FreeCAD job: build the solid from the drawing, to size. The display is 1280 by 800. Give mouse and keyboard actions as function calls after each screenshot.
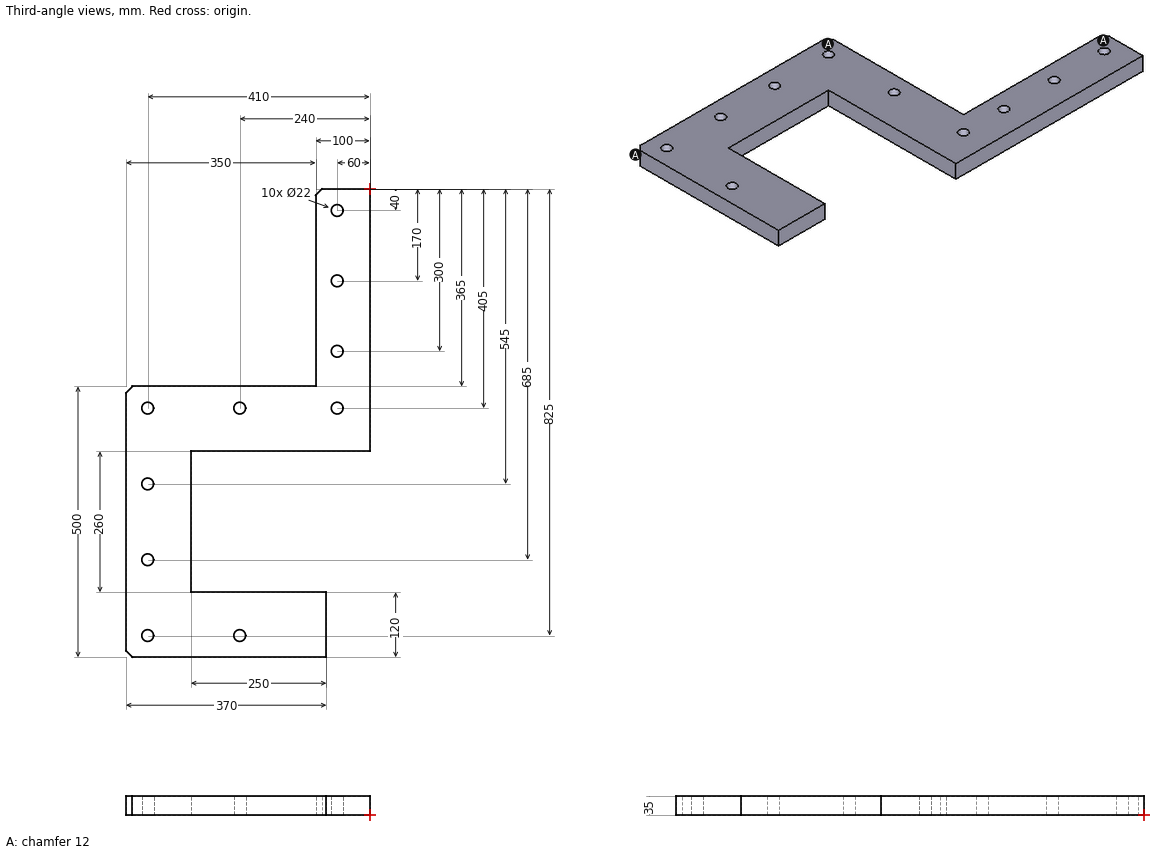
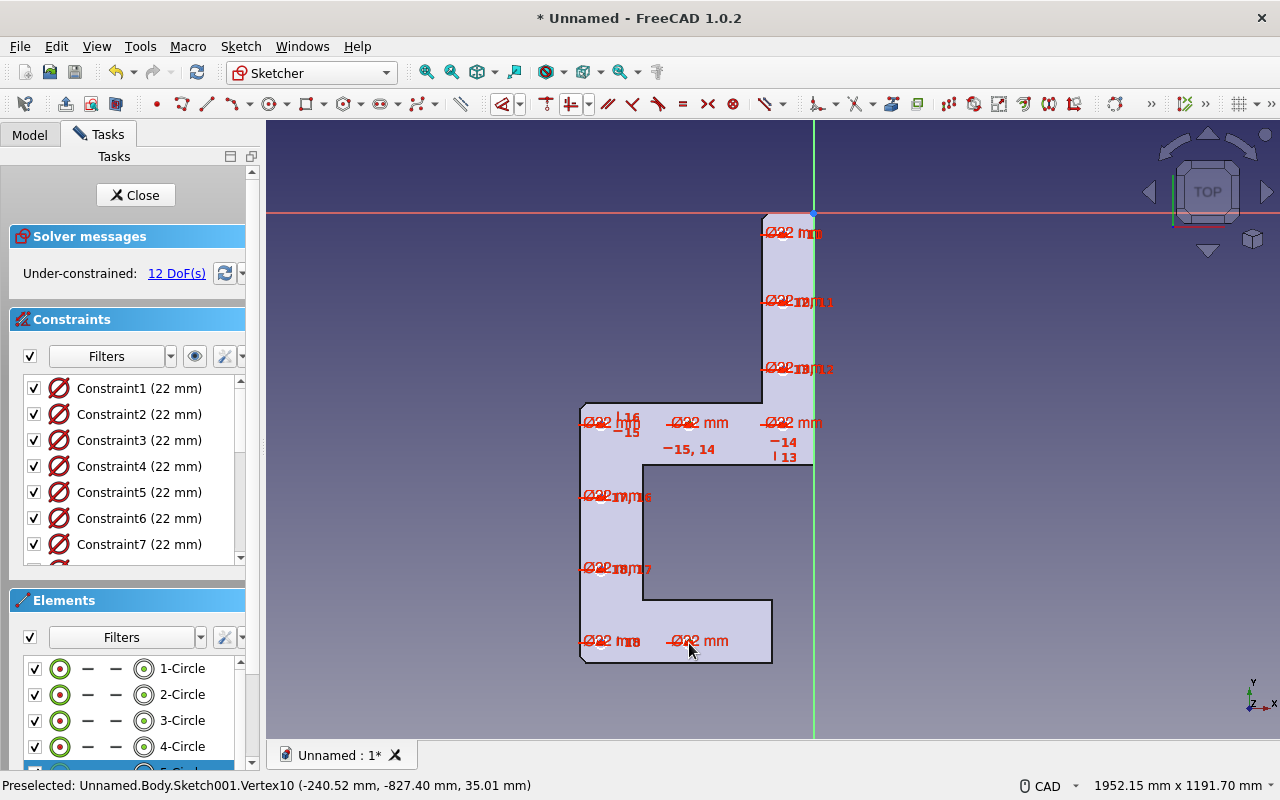
click(588, 104)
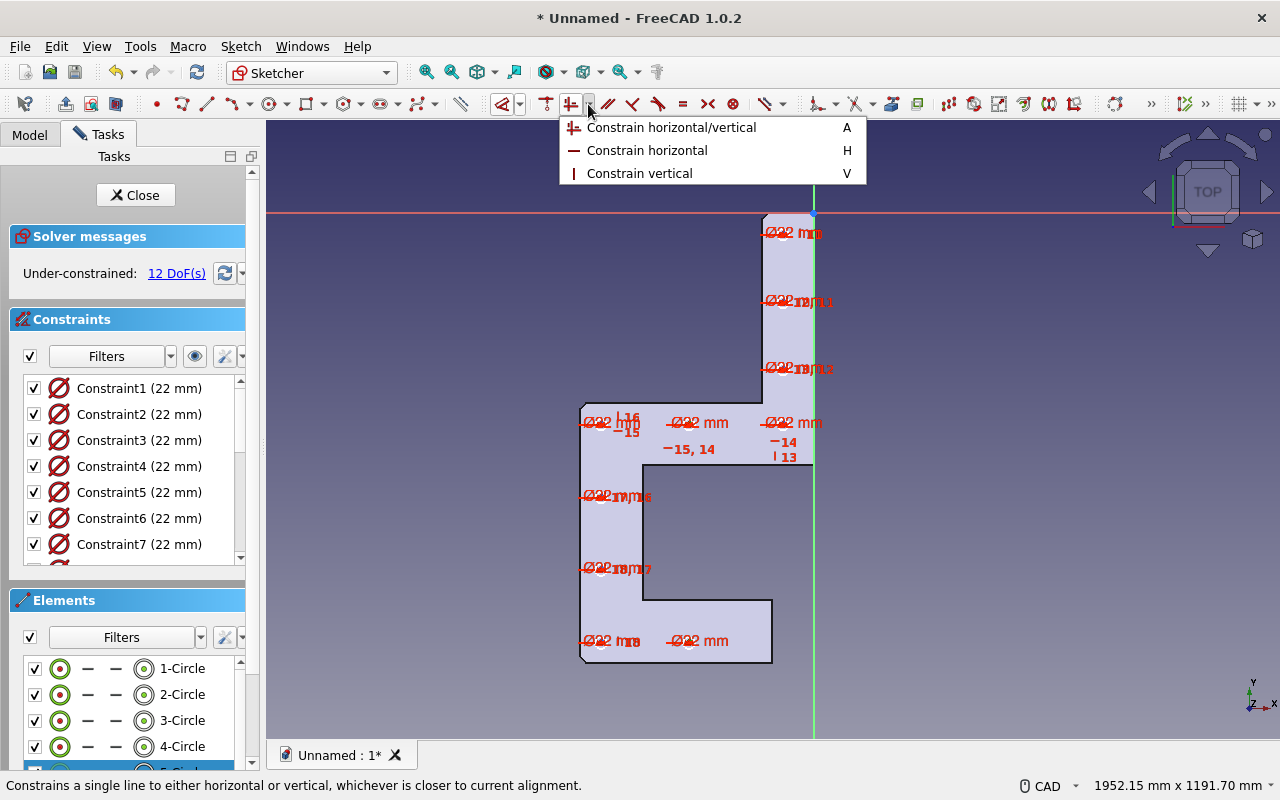
click(713, 174)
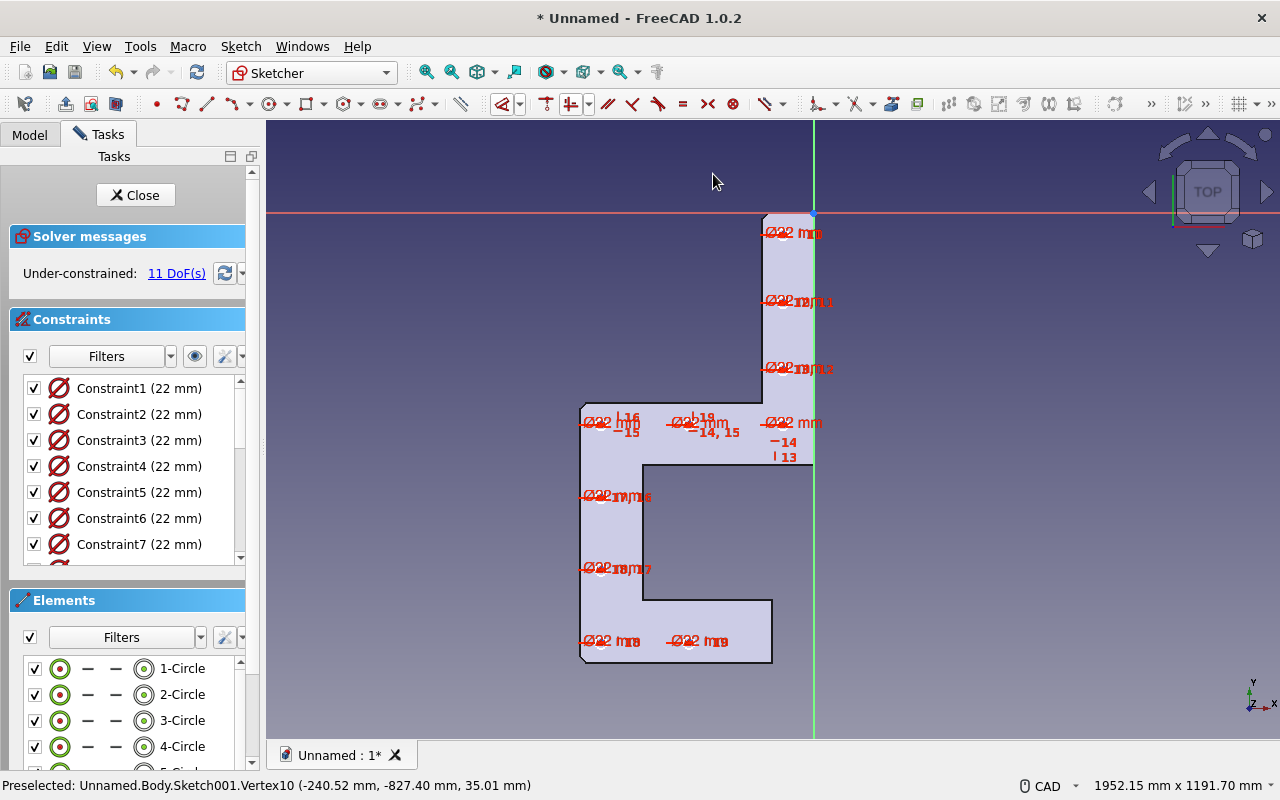
click(601, 643)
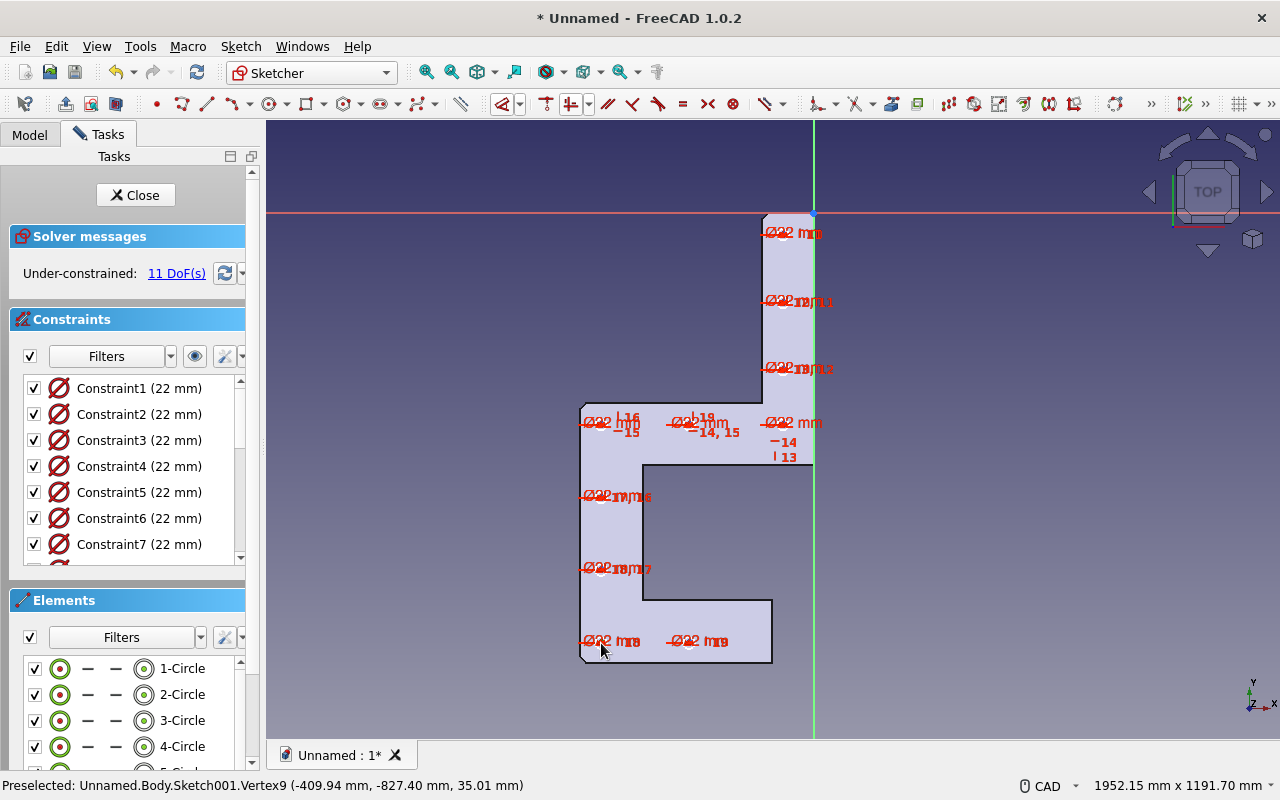
click(689, 643)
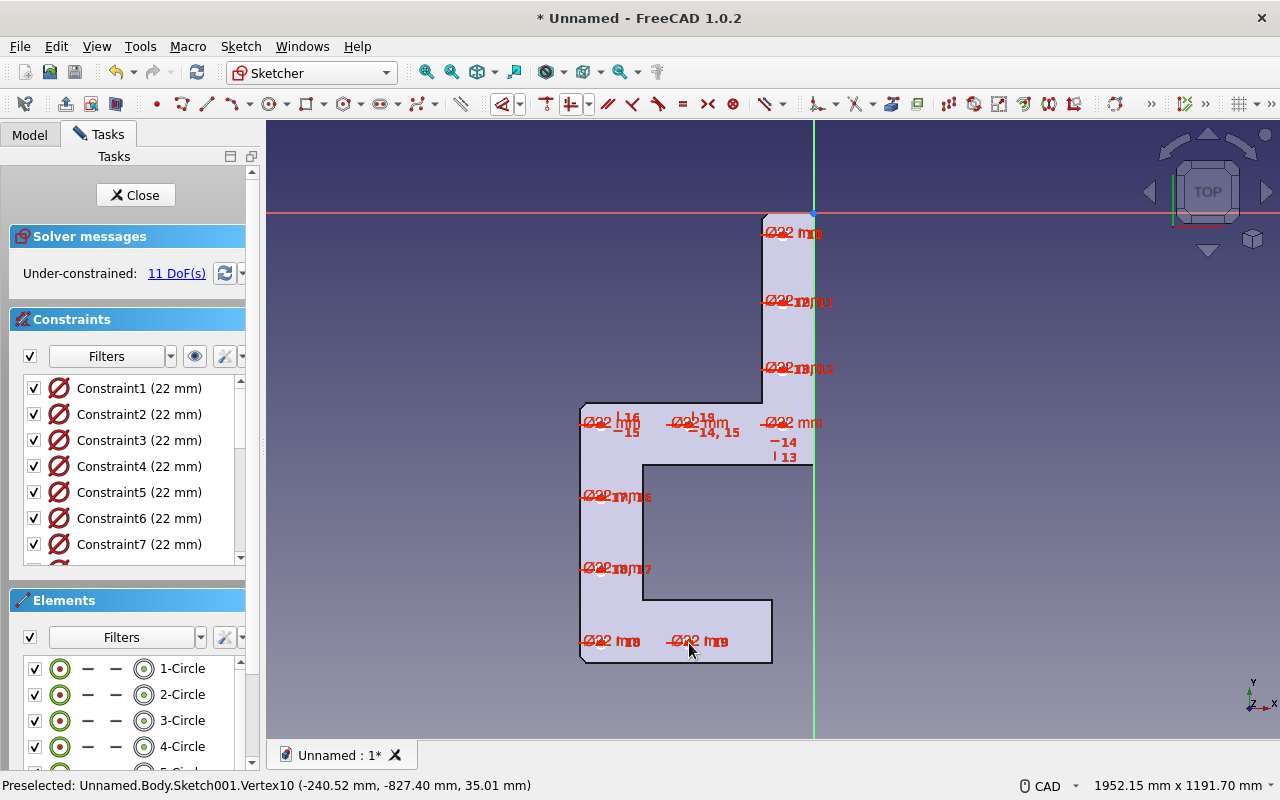
click(588, 104)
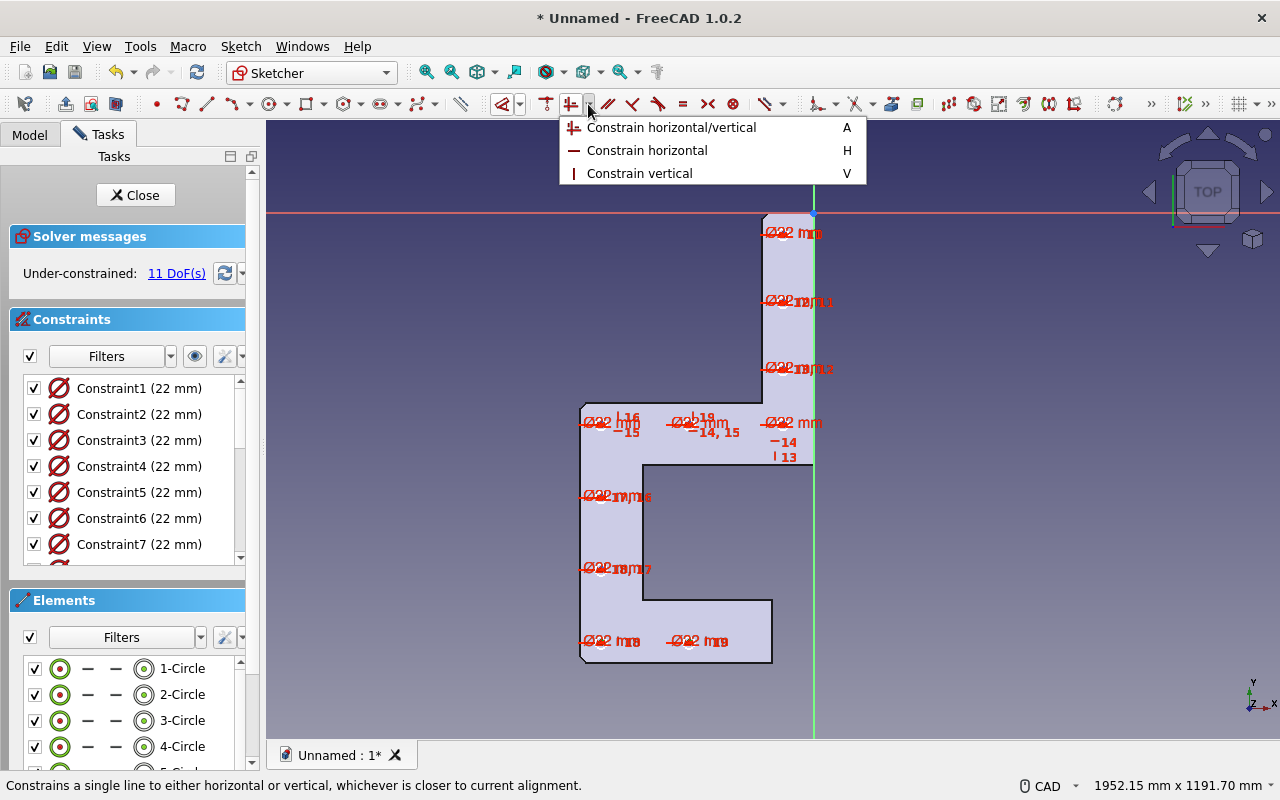
click(713, 150)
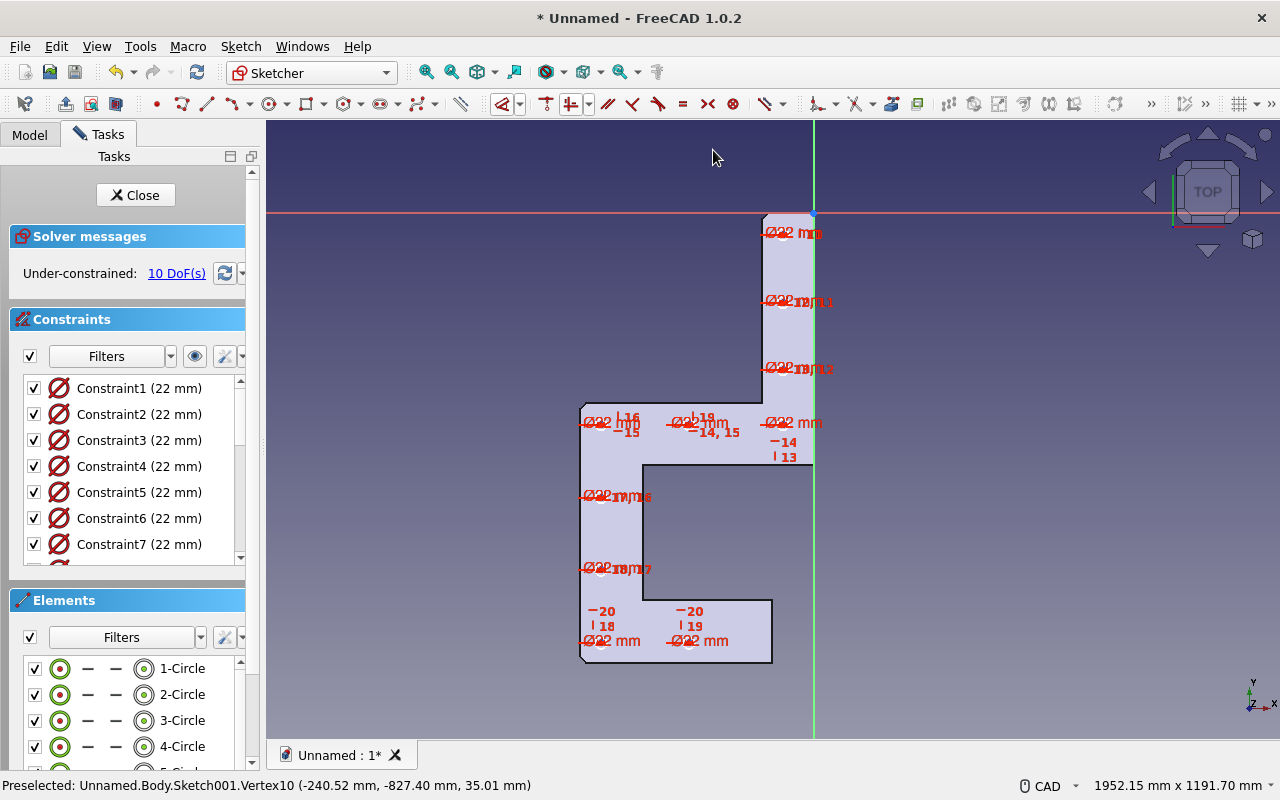
scroll(783, 235, up, 2)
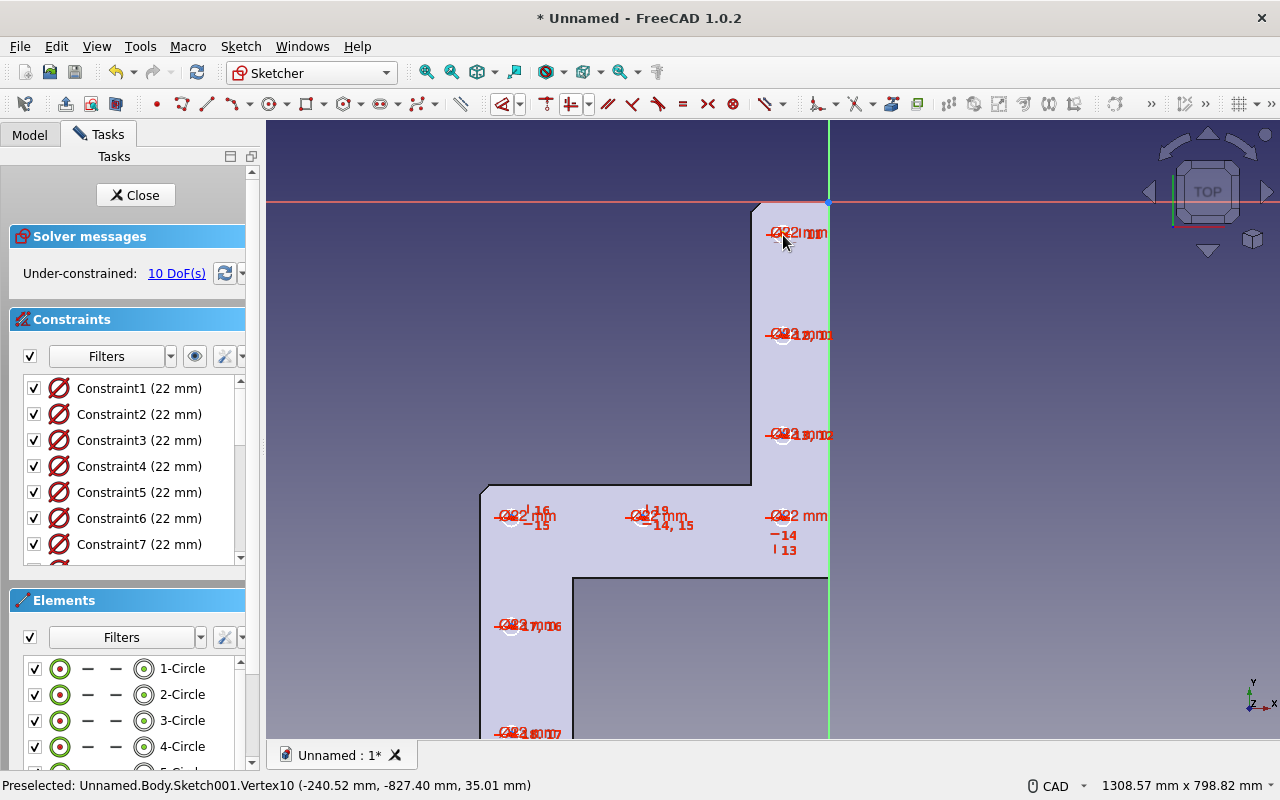
click(783, 235)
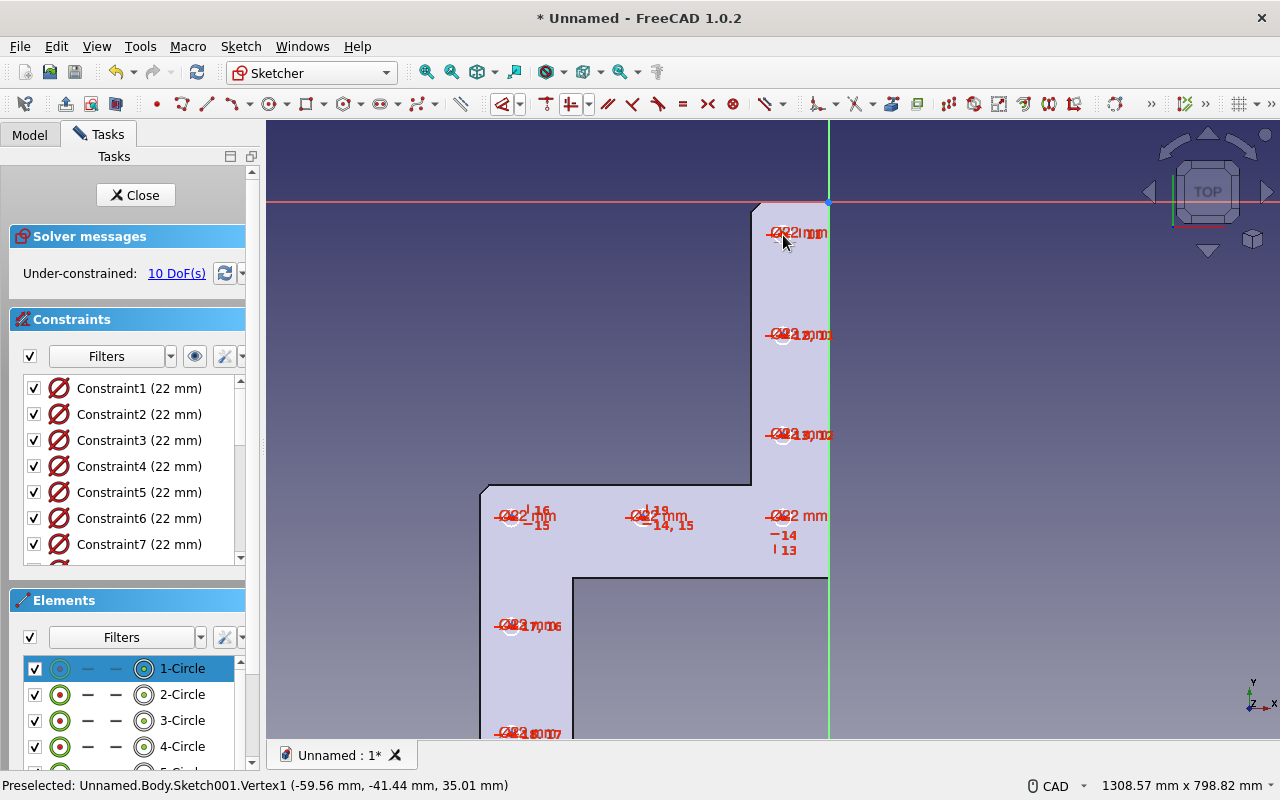
click(520, 104)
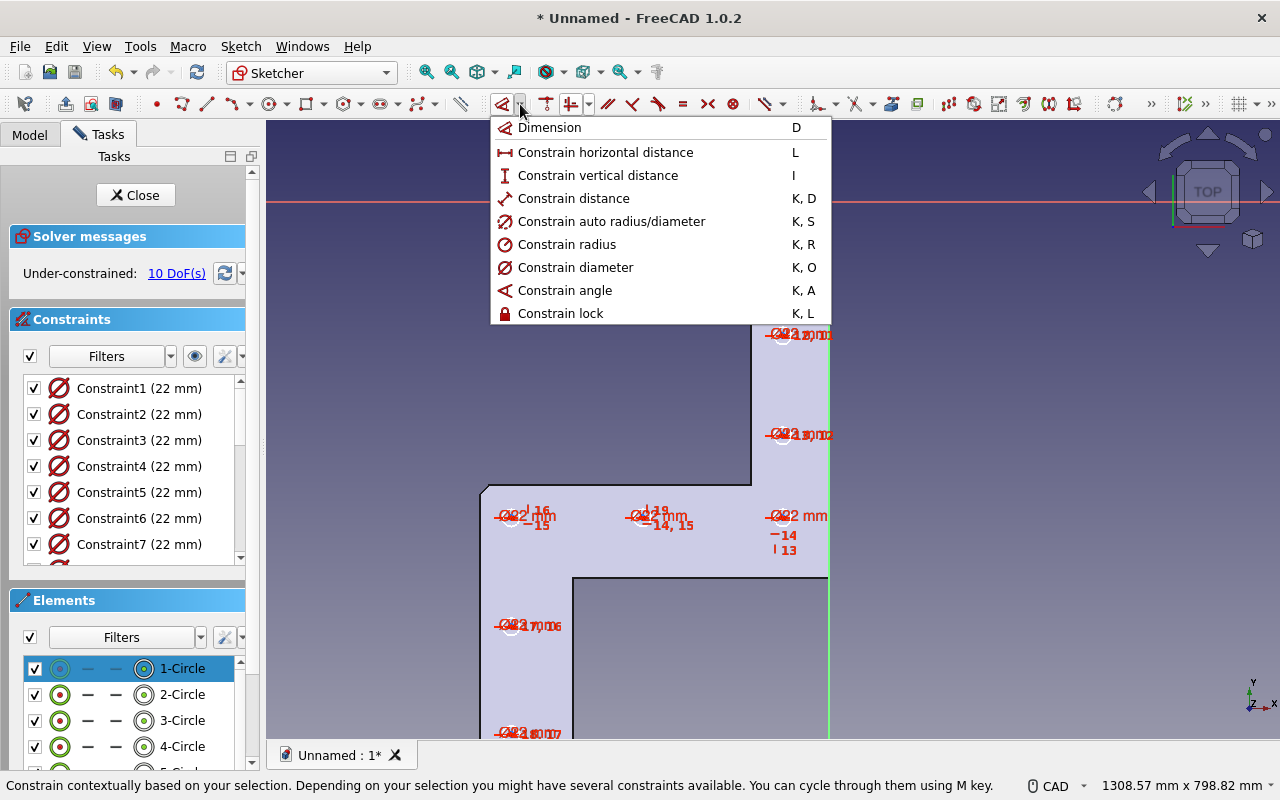
click(661, 152)